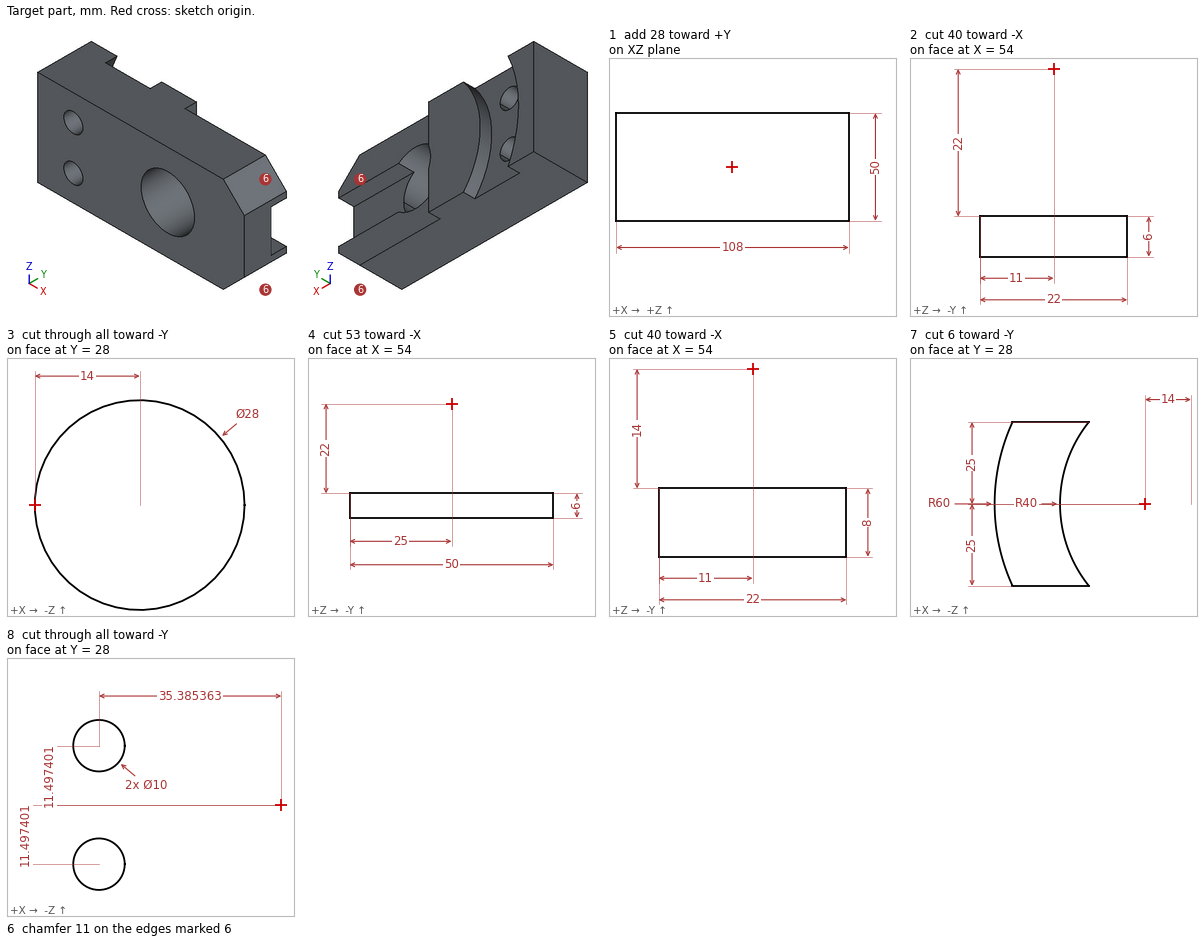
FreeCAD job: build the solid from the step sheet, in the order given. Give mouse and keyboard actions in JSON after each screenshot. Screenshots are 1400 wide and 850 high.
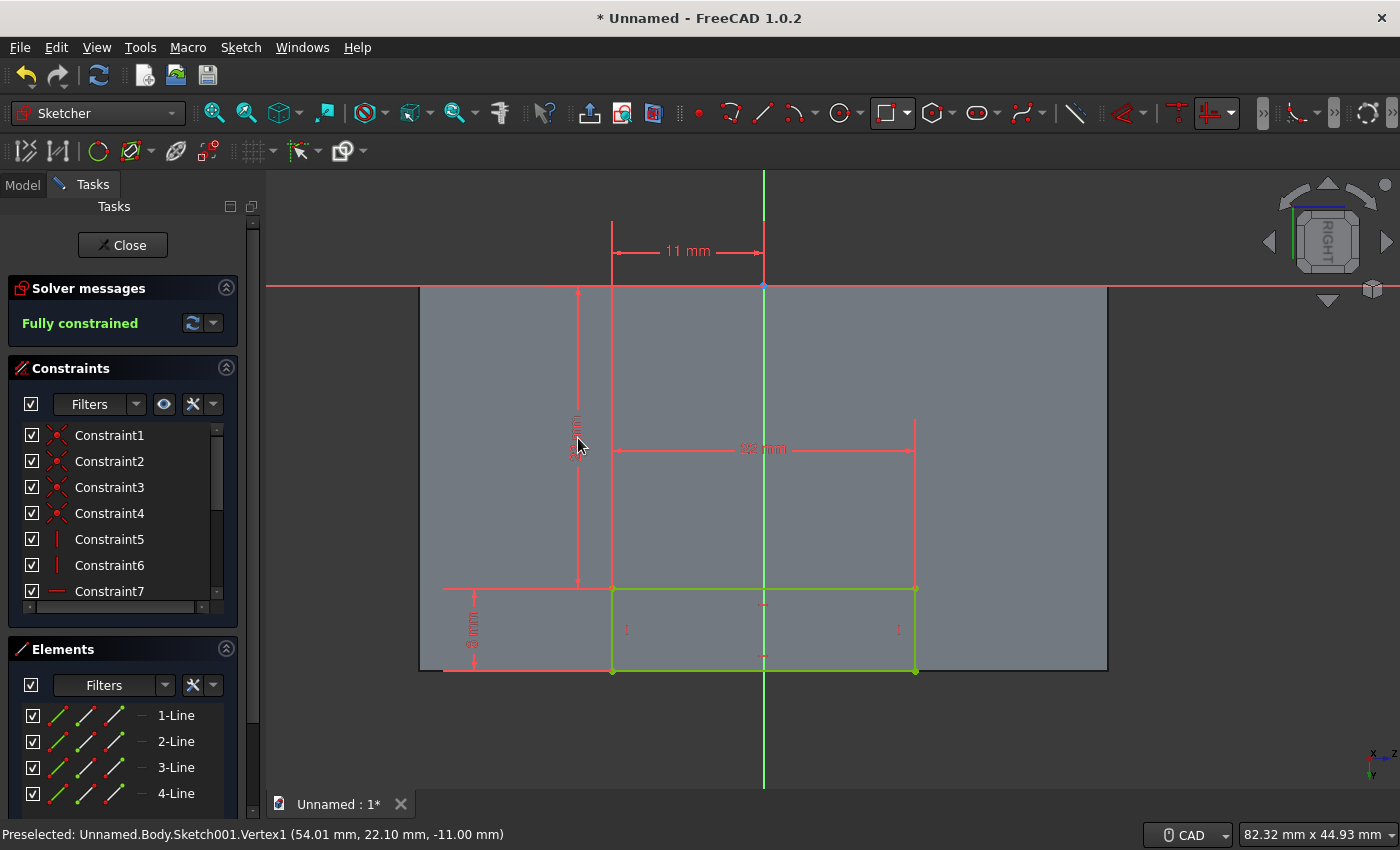
{"action": "left_click", "coordinate": [123, 245]}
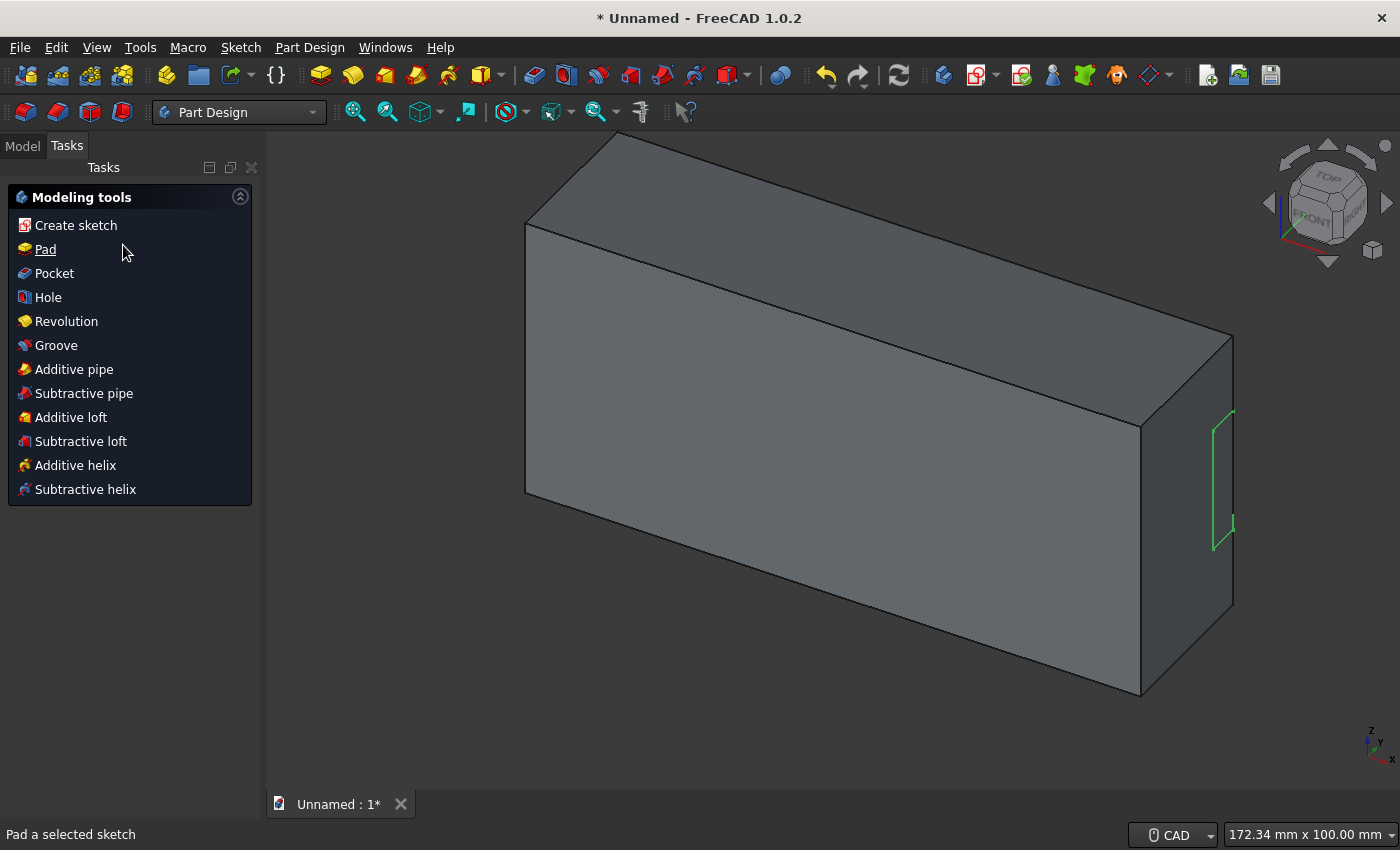
{"action": "left_click", "coordinate": [536, 76]}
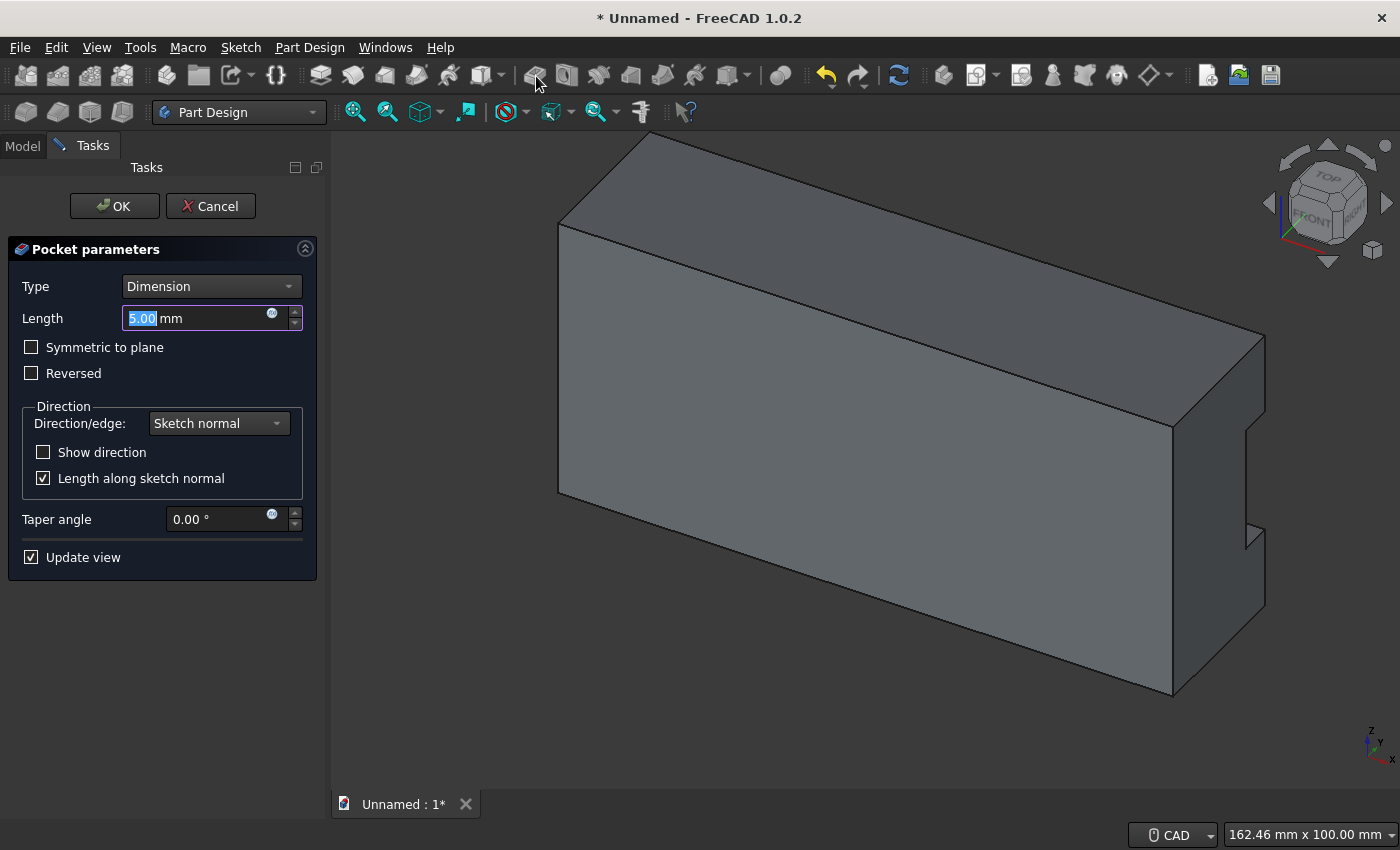
{"action": "type", "text": "40"}
{"action": "key", "text": "Tab"}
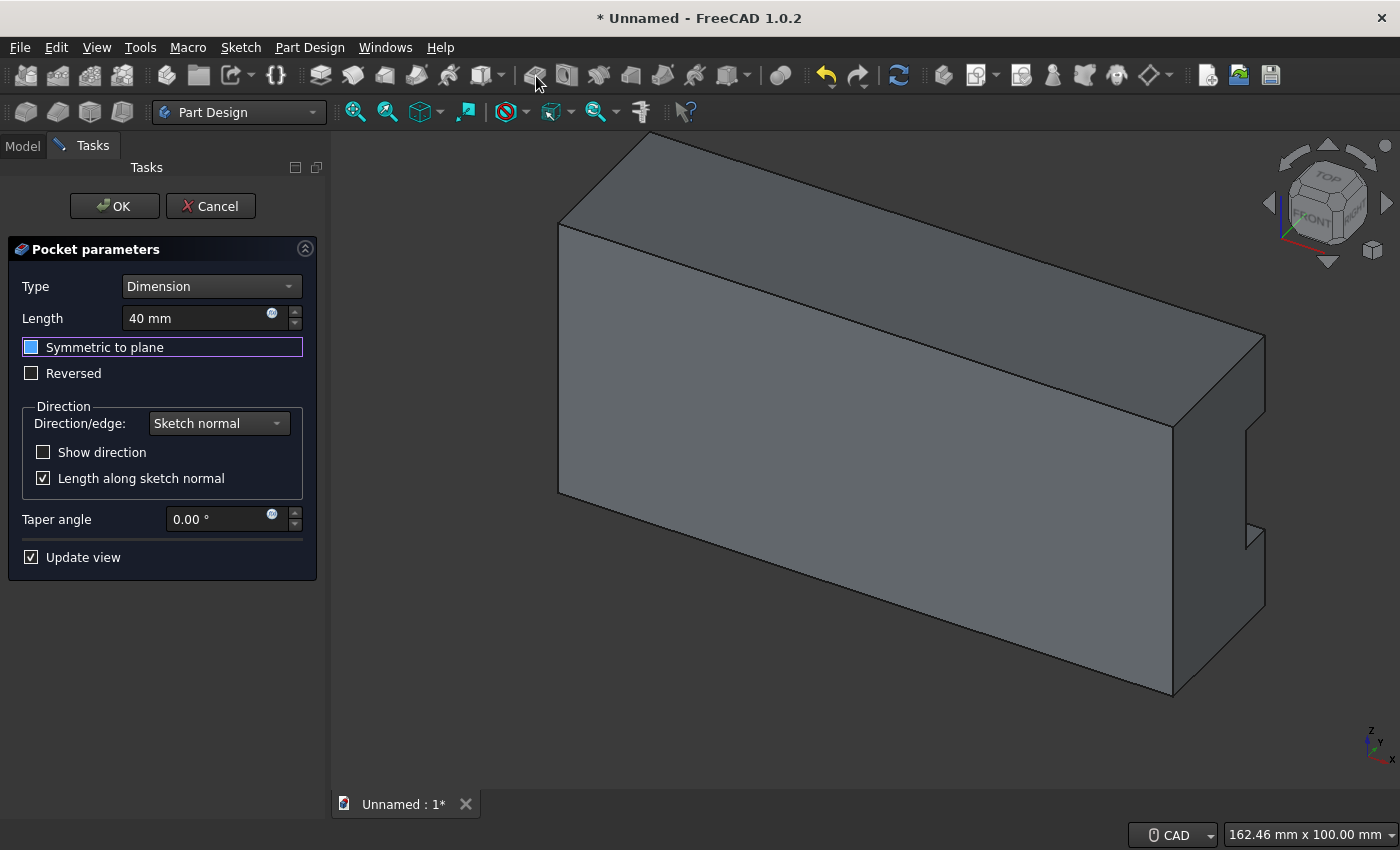
{"action": "left_click", "coordinate": [115, 206]}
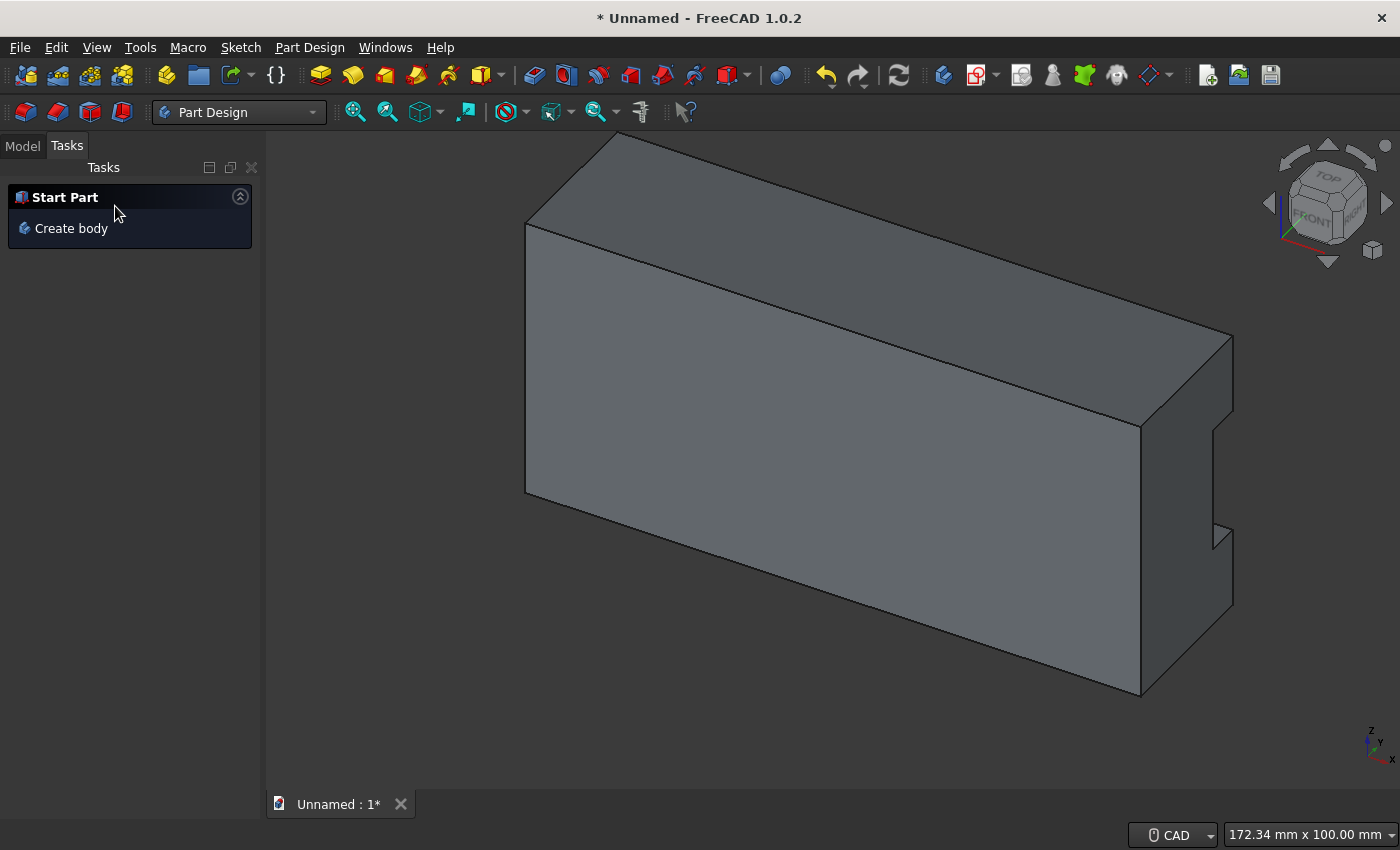
{"action": "key", "text": "4"}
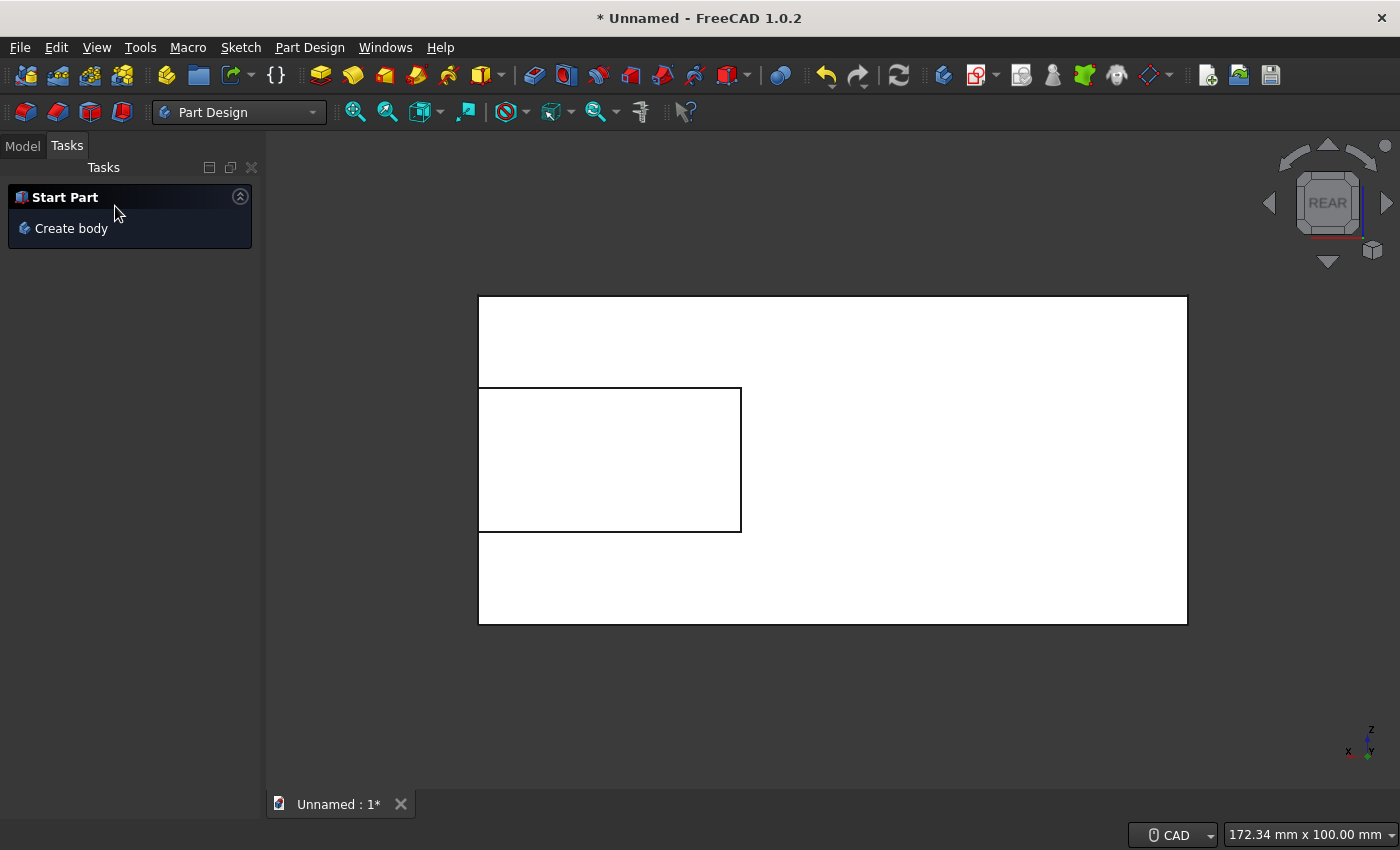
{"action": "left_click", "coordinate": [935, 459]}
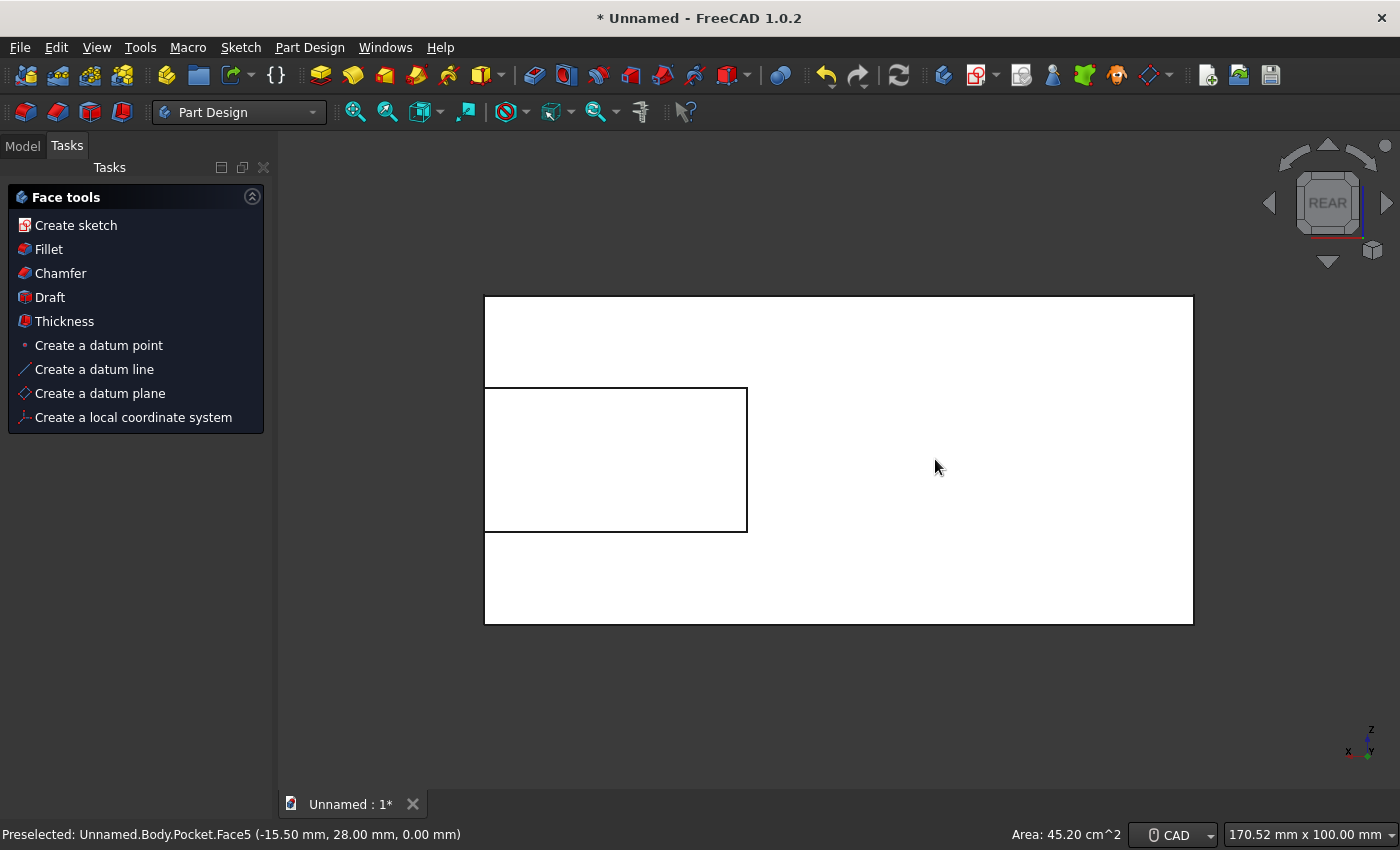
{"action": "left_click", "coordinate": [976, 76]}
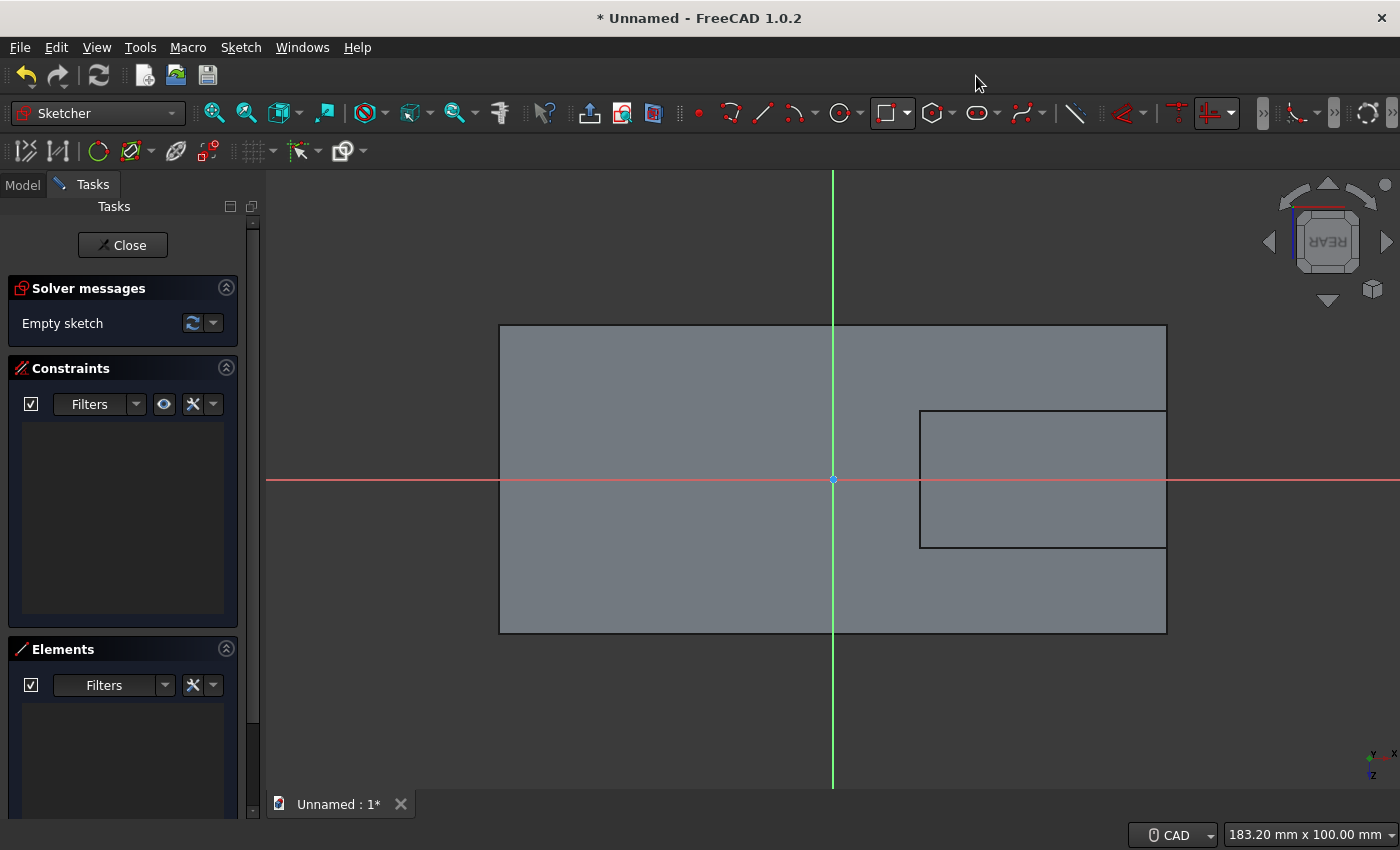
{"action": "scroll", "coordinate": [1046, 480], "scroll_direction": "up", "scroll_amount": 4}